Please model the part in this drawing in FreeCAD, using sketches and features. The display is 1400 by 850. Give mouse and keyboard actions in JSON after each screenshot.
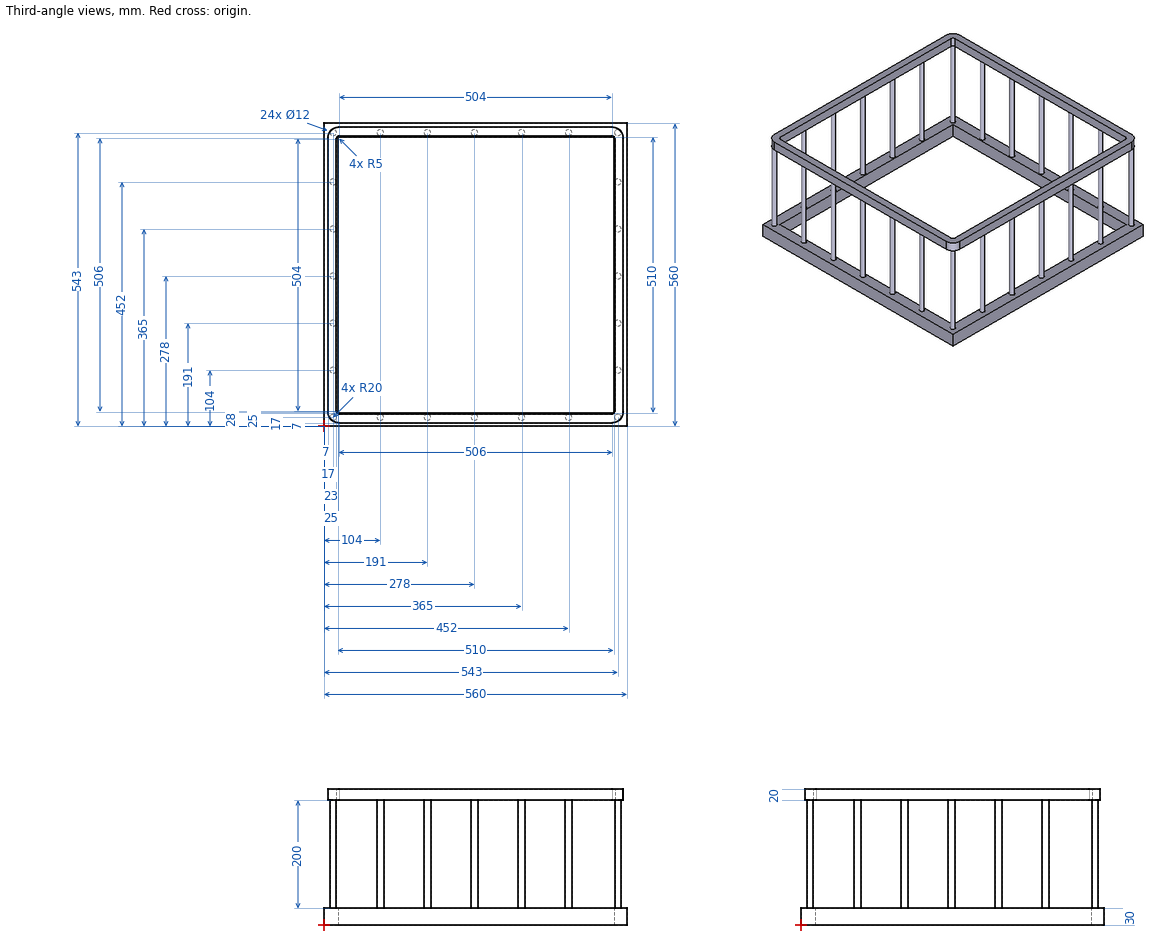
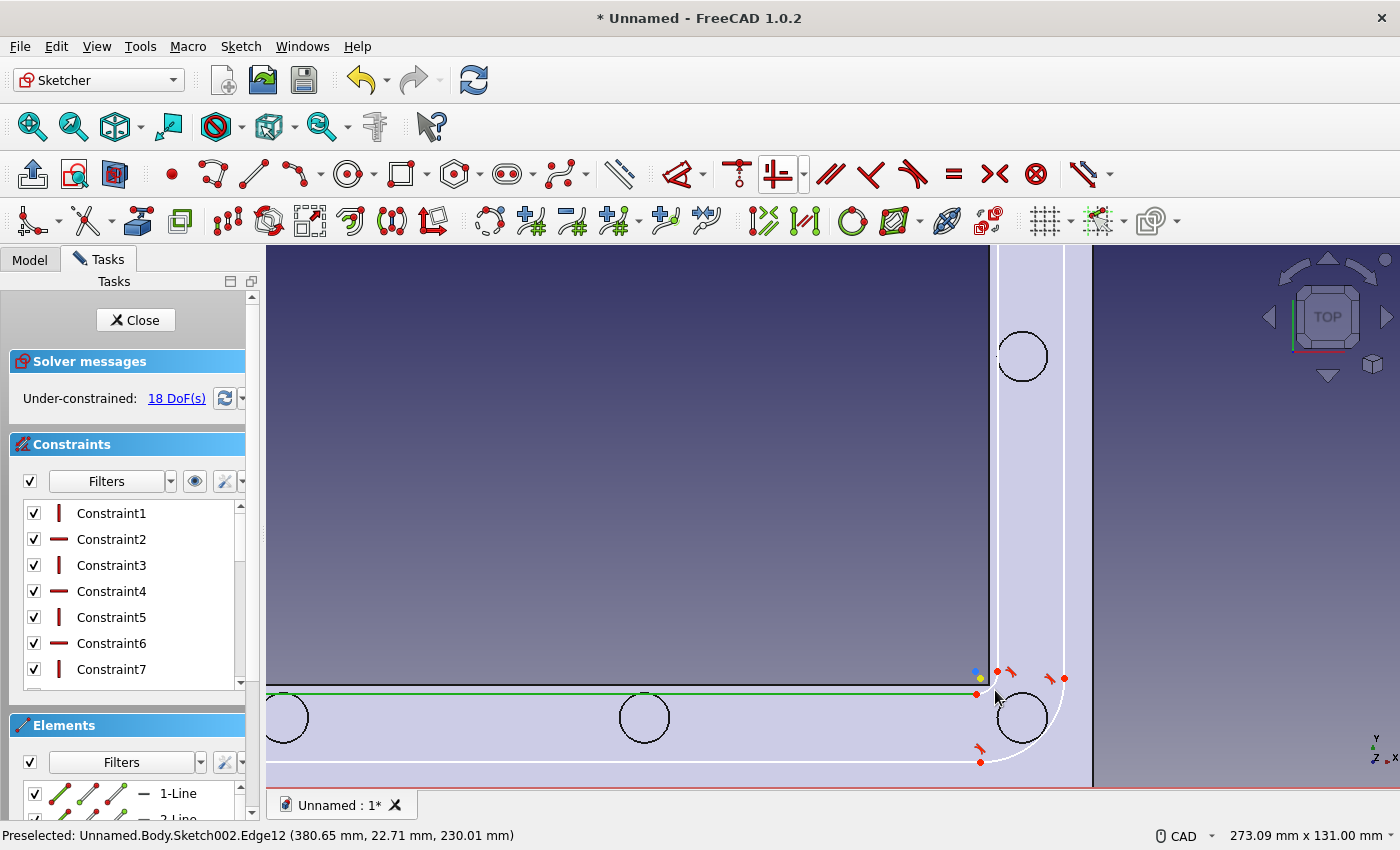
{"action": "left_click", "coordinate": [992, 687]}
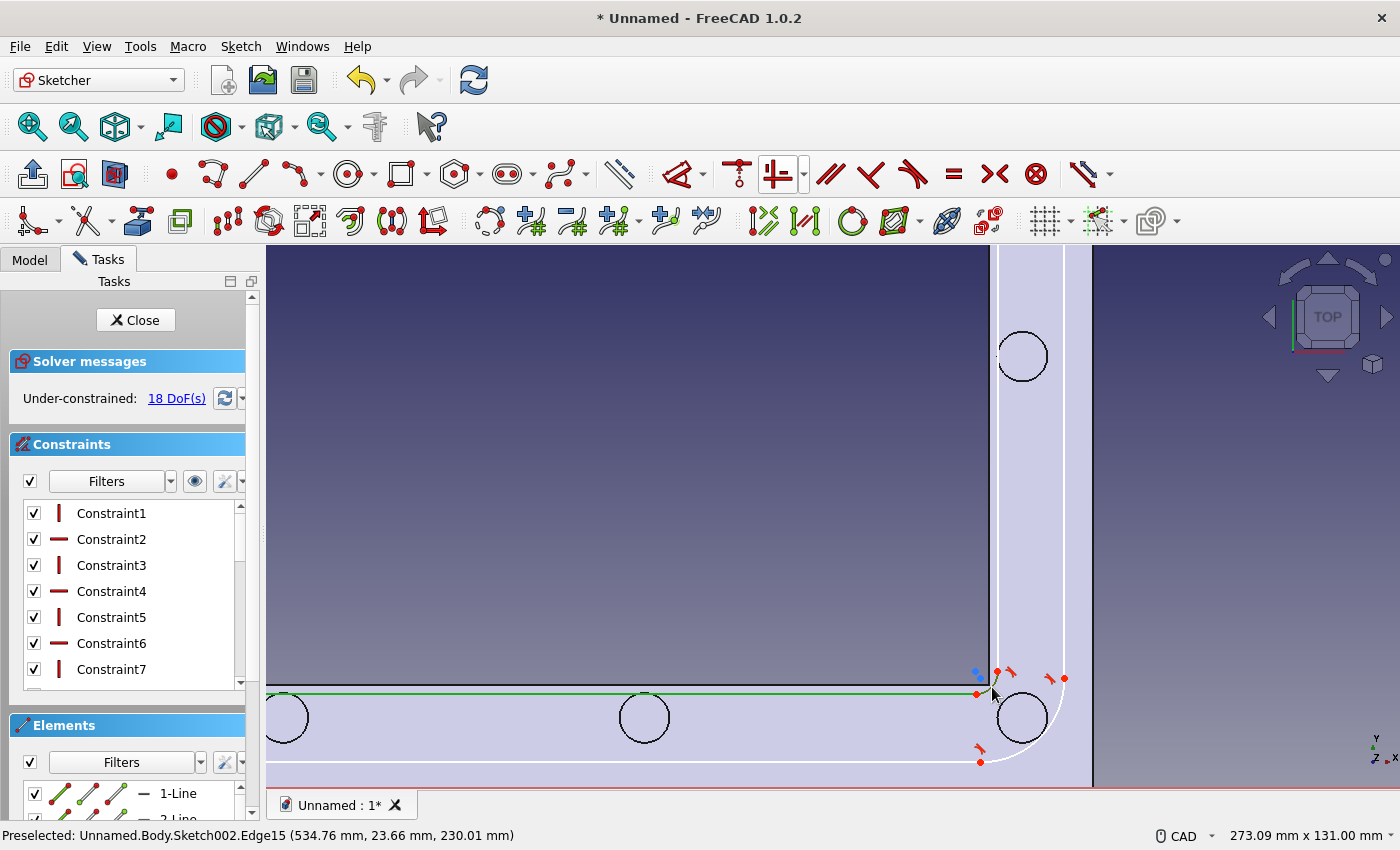
{"action": "left_click", "coordinate": [913, 174]}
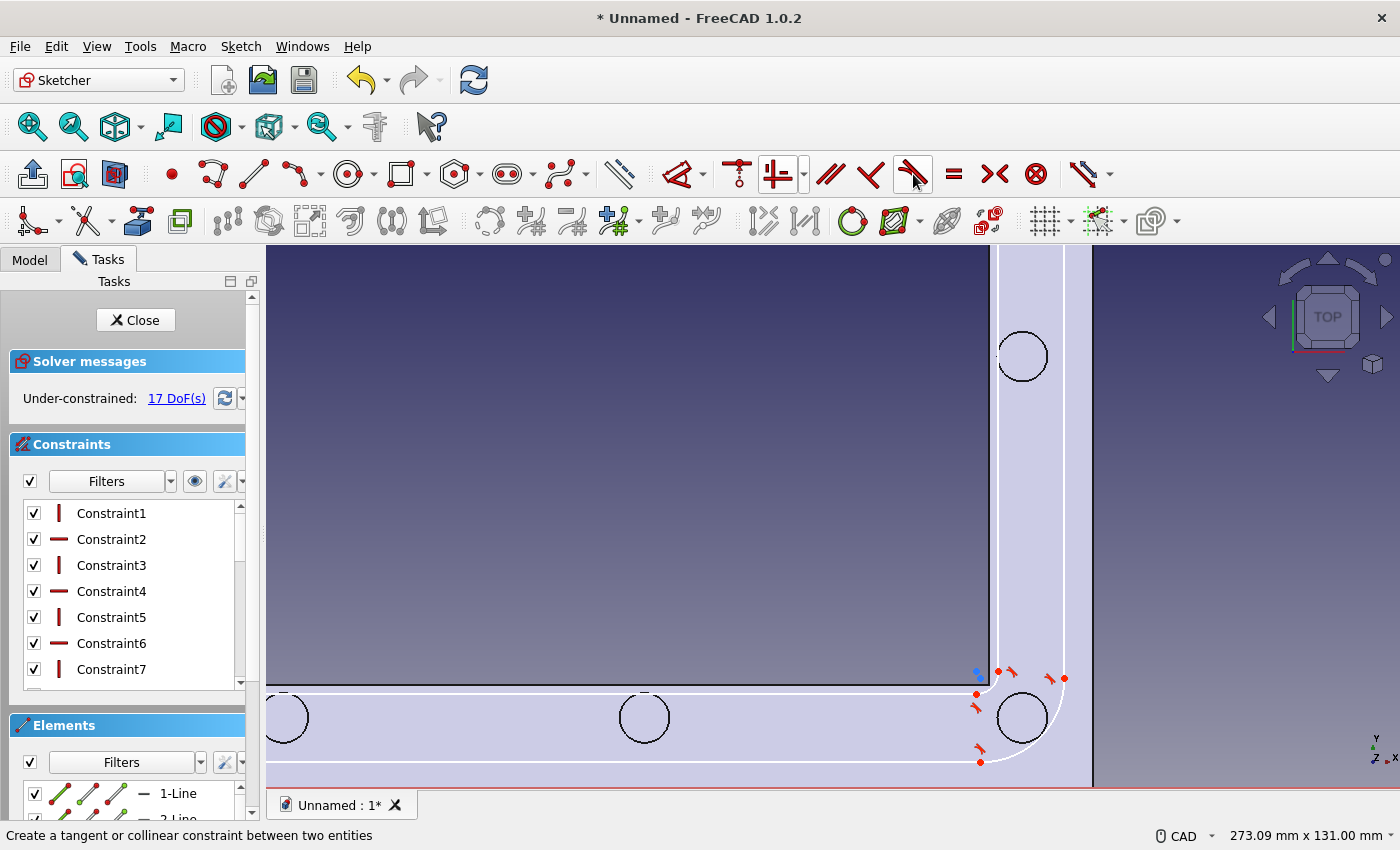
{"action": "scroll", "coordinate": [933, 691], "scroll_direction": "down", "scroll_amount": 9}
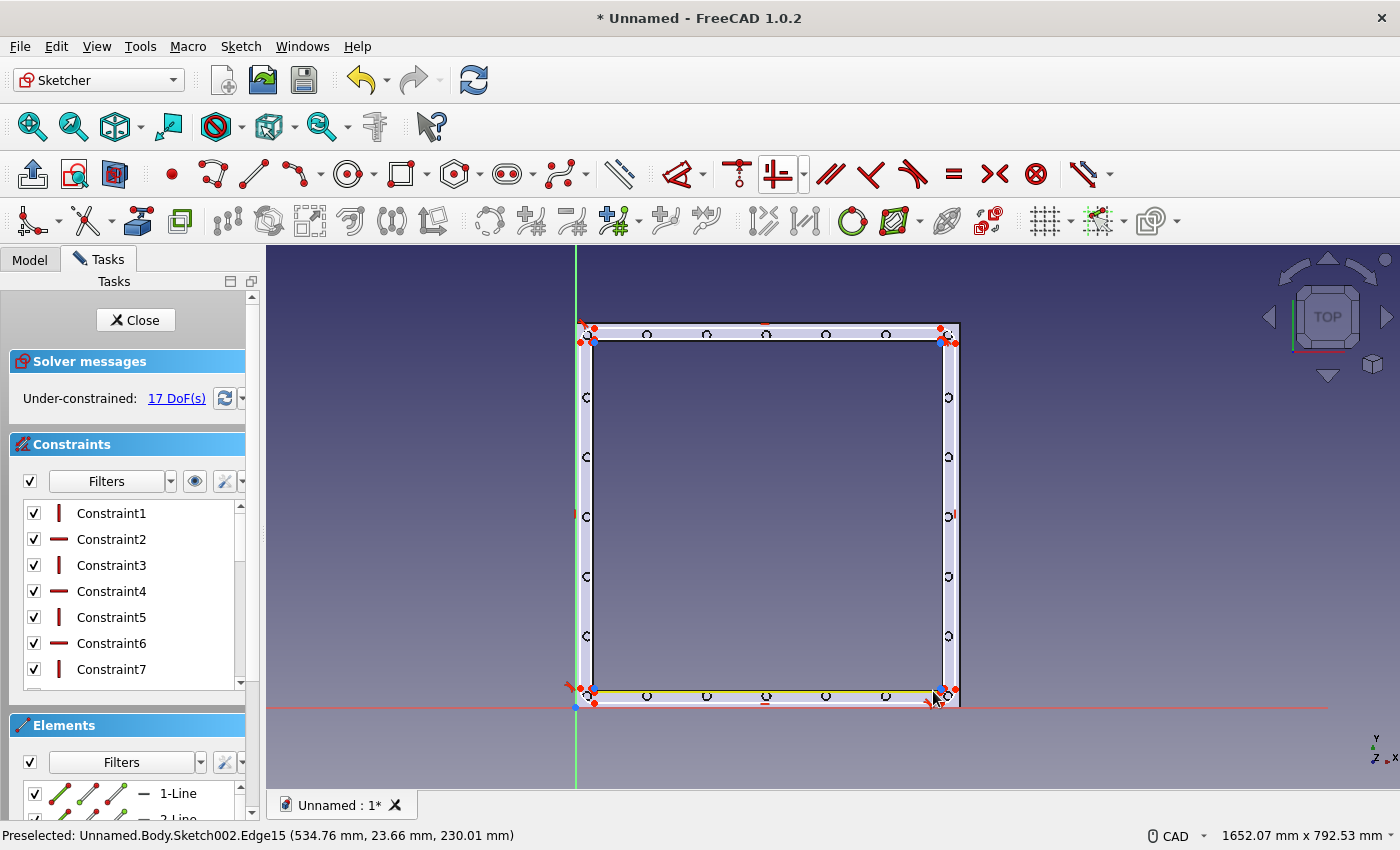
{"action": "scroll", "coordinate": [837, 692], "scroll_direction": "up", "scroll_amount": 2}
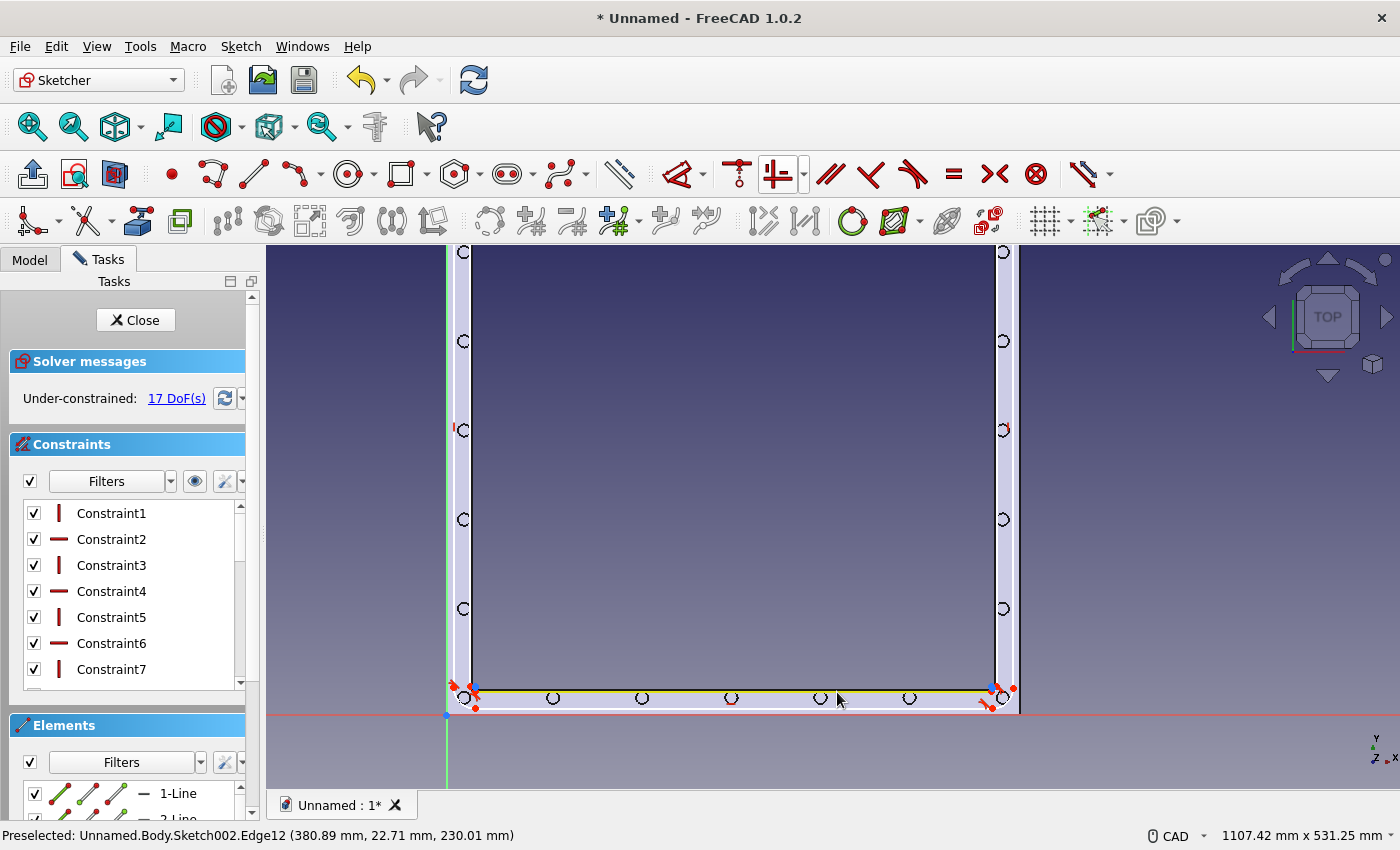
{"action": "left_click", "coordinate": [837, 692]}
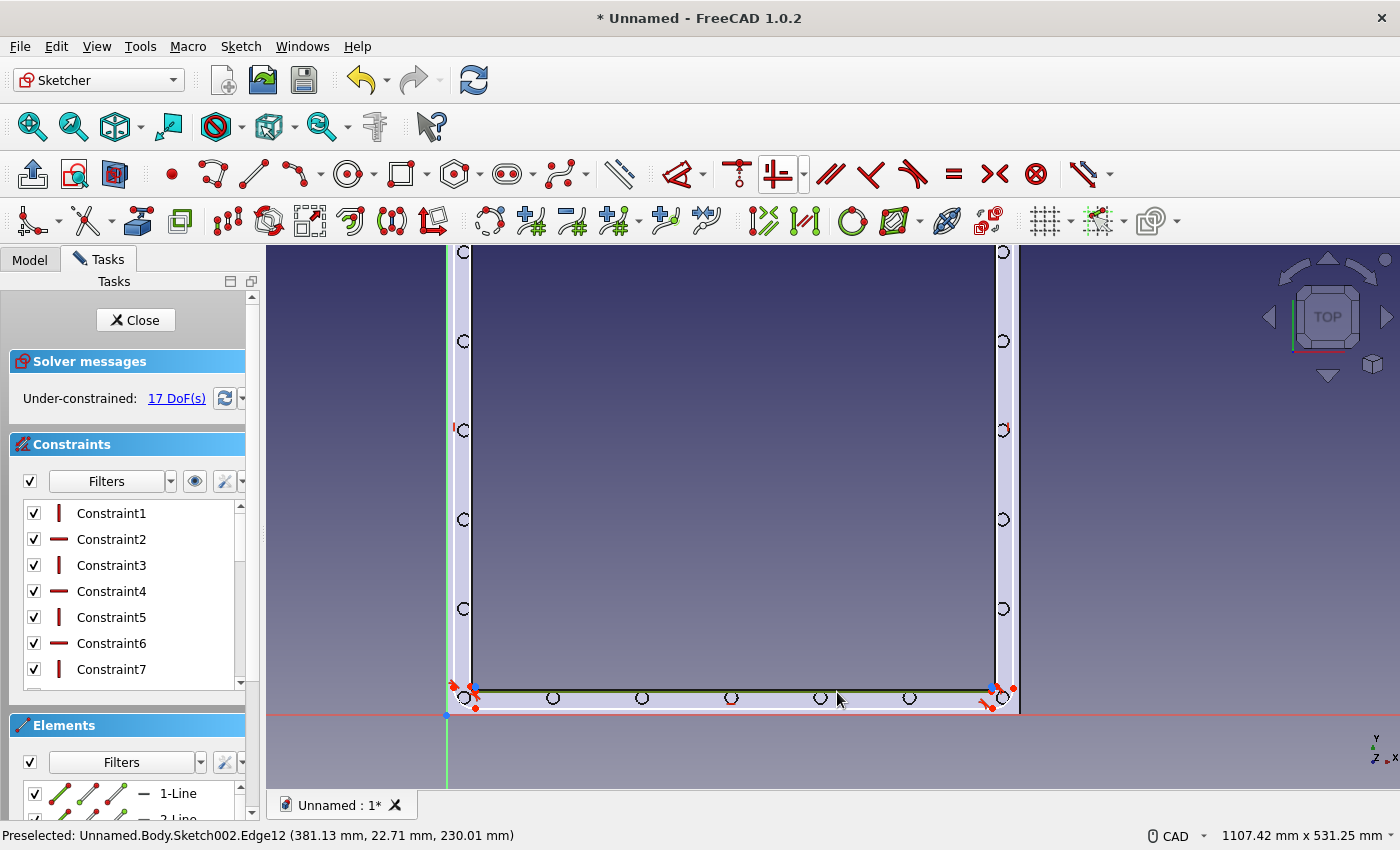
{"action": "scroll", "coordinate": [472, 690], "scroll_direction": "up", "scroll_amount": 7}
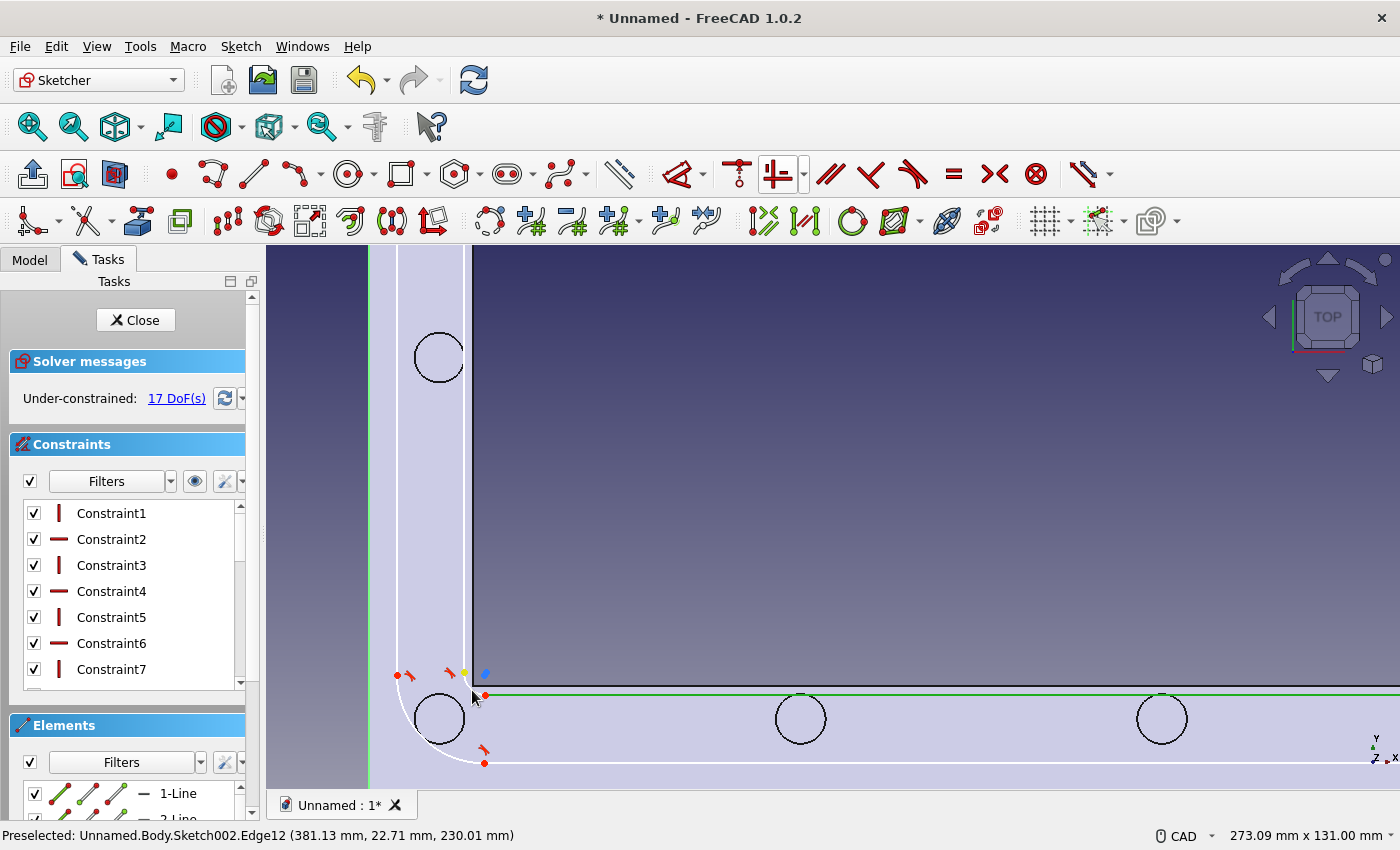
{"action": "left_click", "coordinate": [470, 688]}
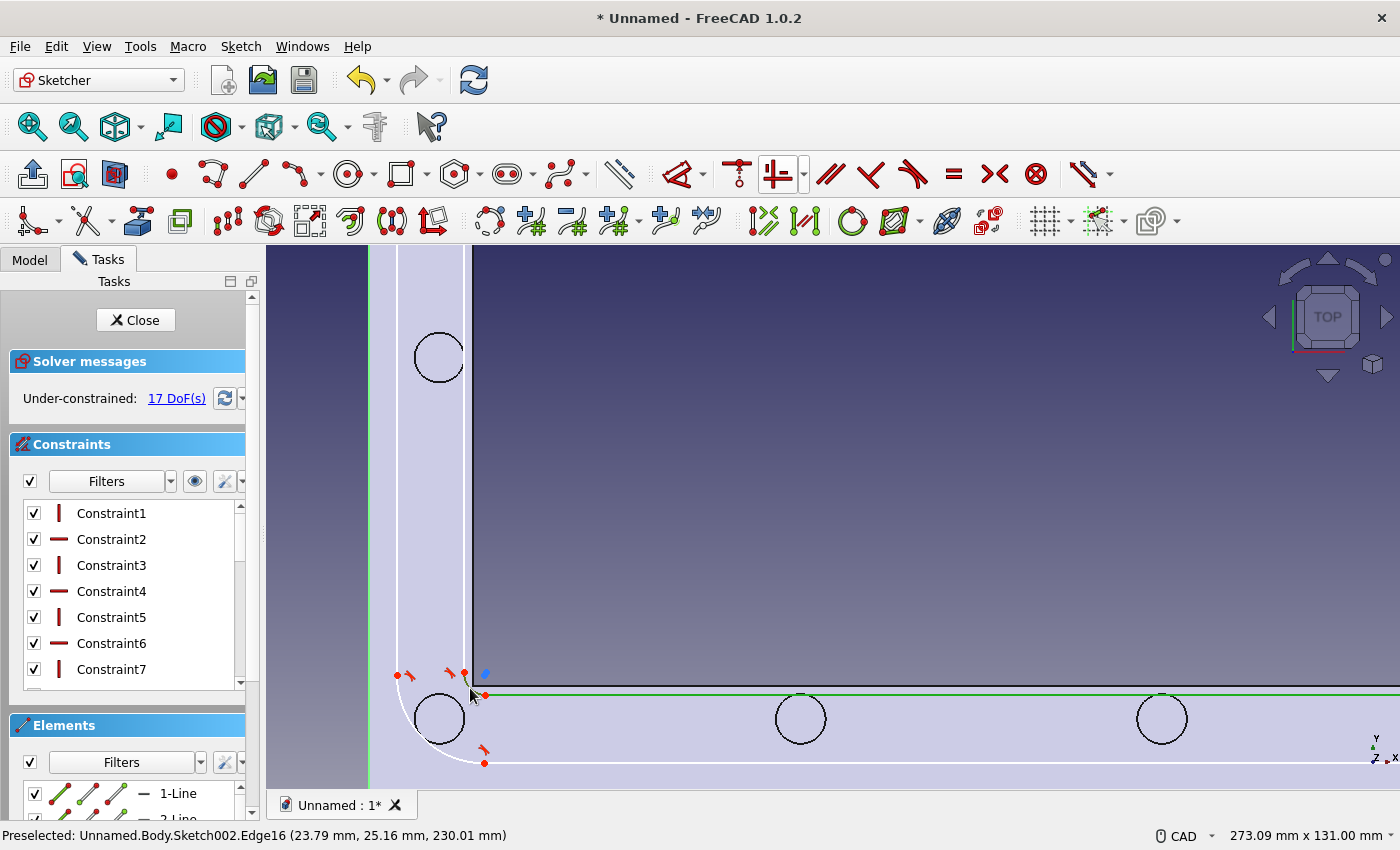
{"action": "left_click", "coordinate": [913, 174]}